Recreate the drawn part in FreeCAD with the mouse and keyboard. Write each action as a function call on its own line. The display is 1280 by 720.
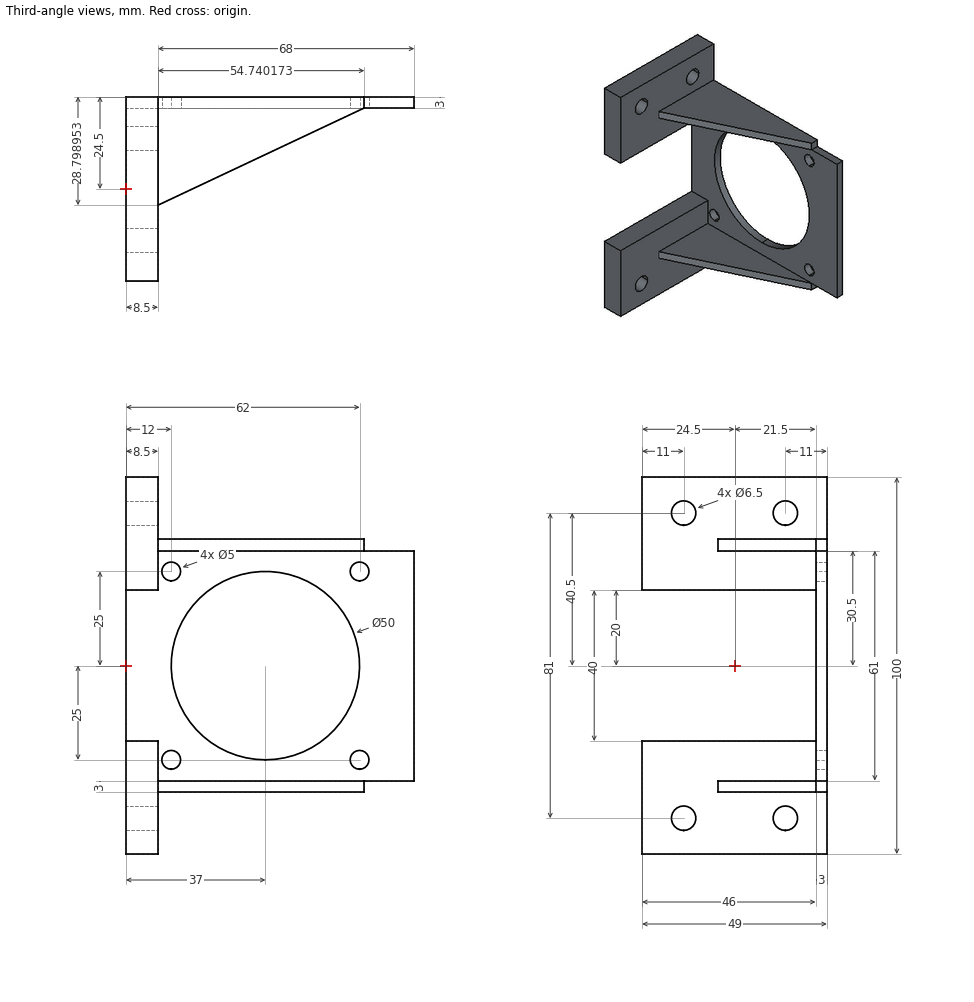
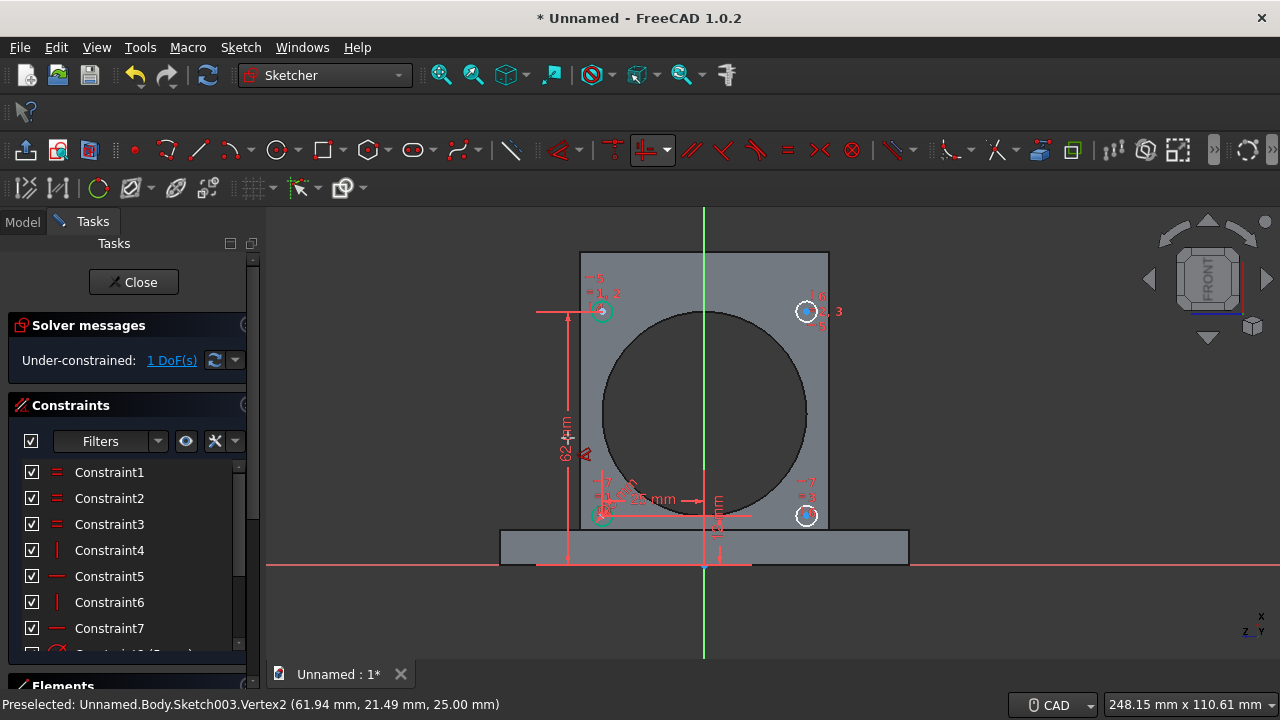
click(807, 312)
click(756, 599)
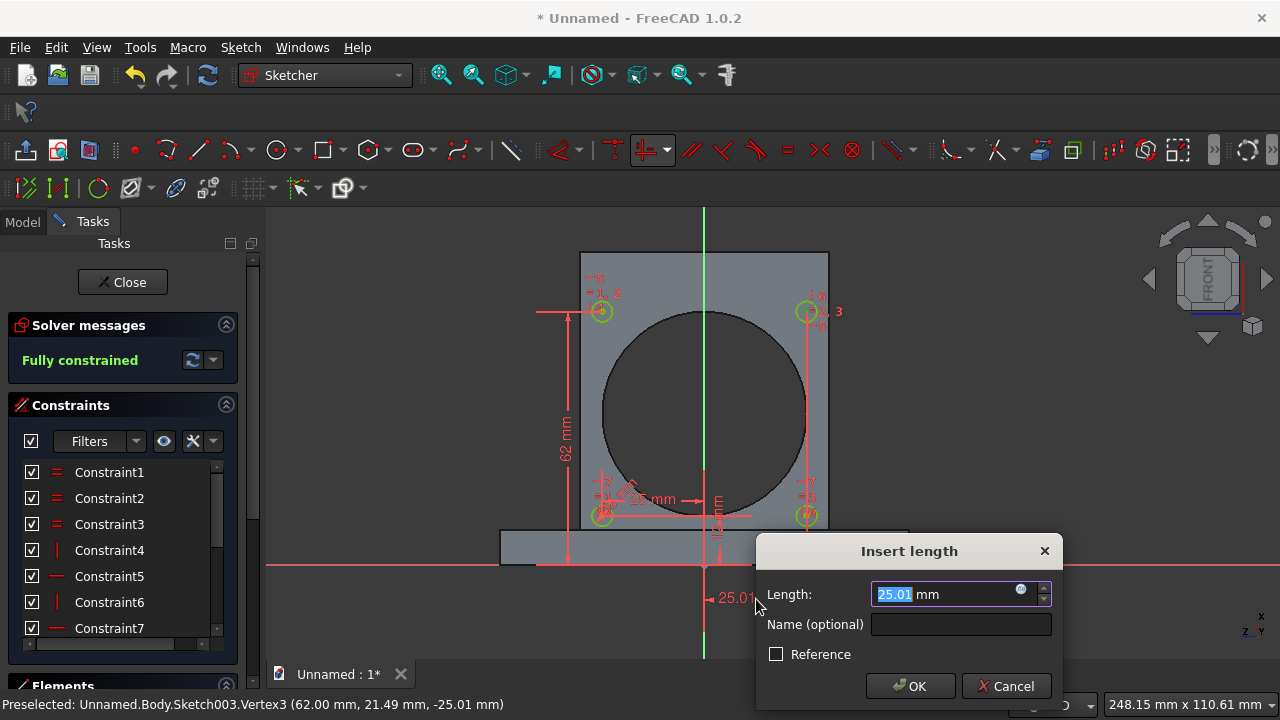
text(25)
key(Return)
key(Escape)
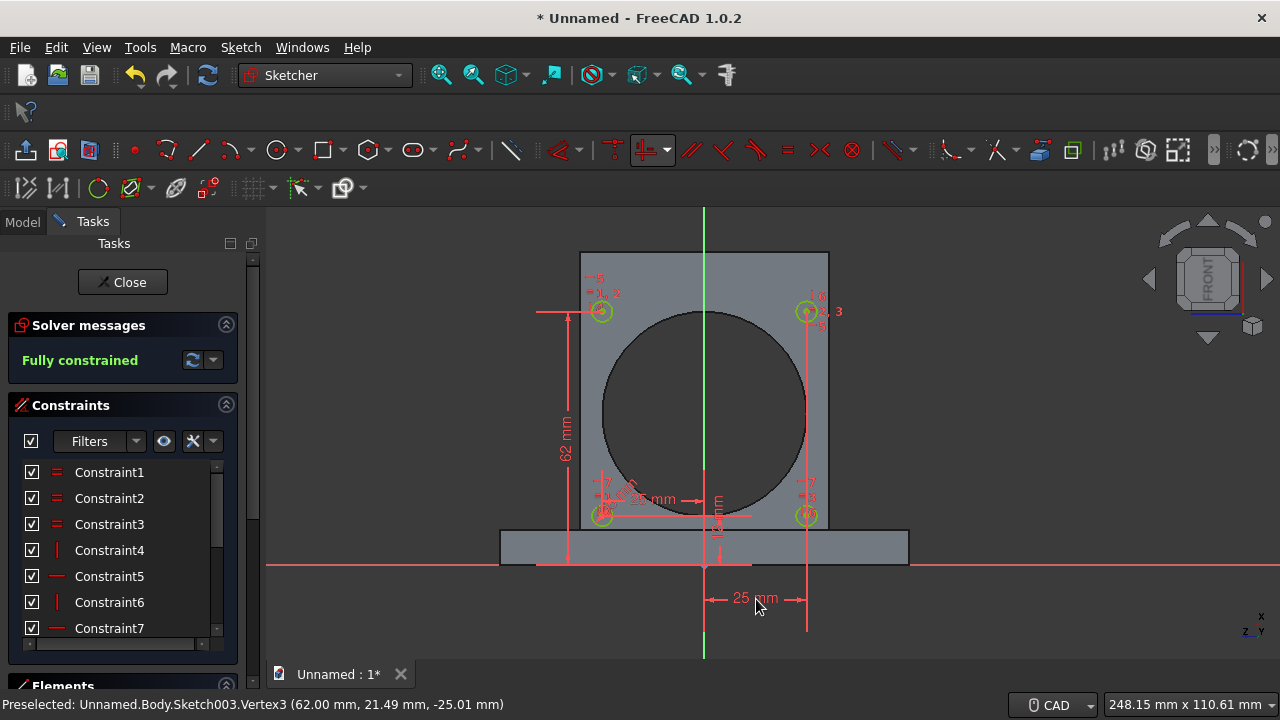
click(123, 282)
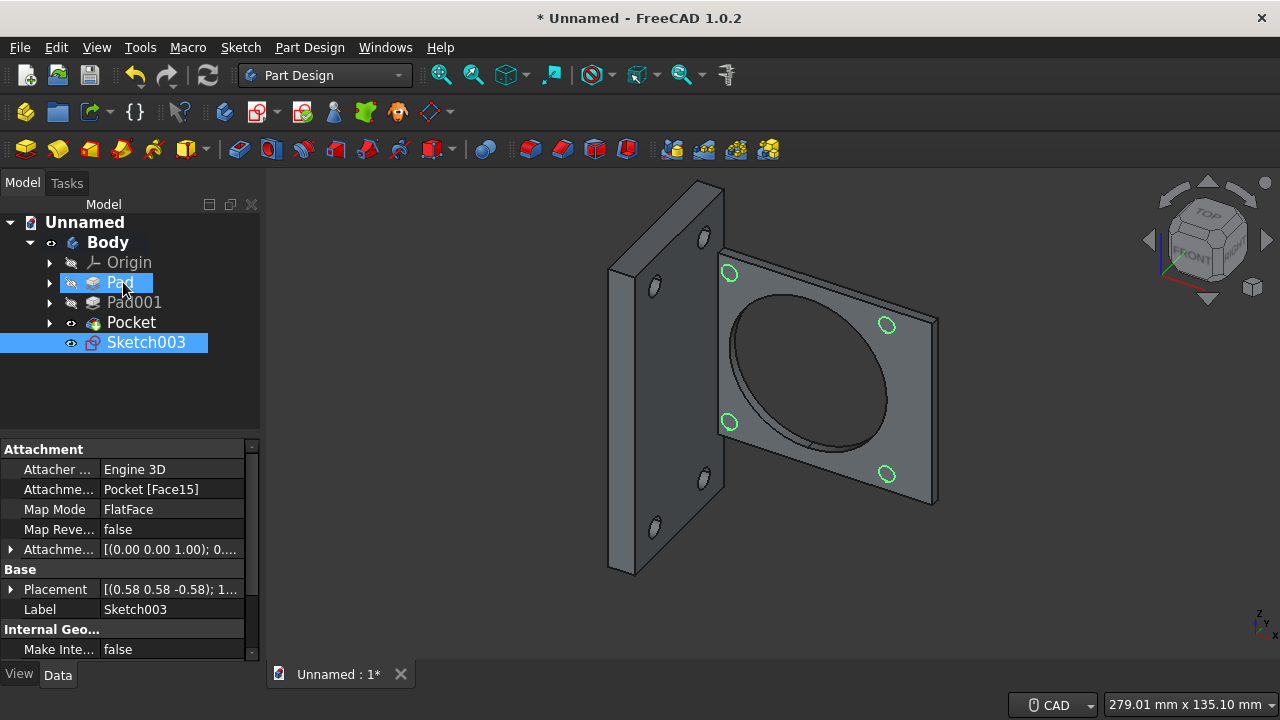
click(240, 150)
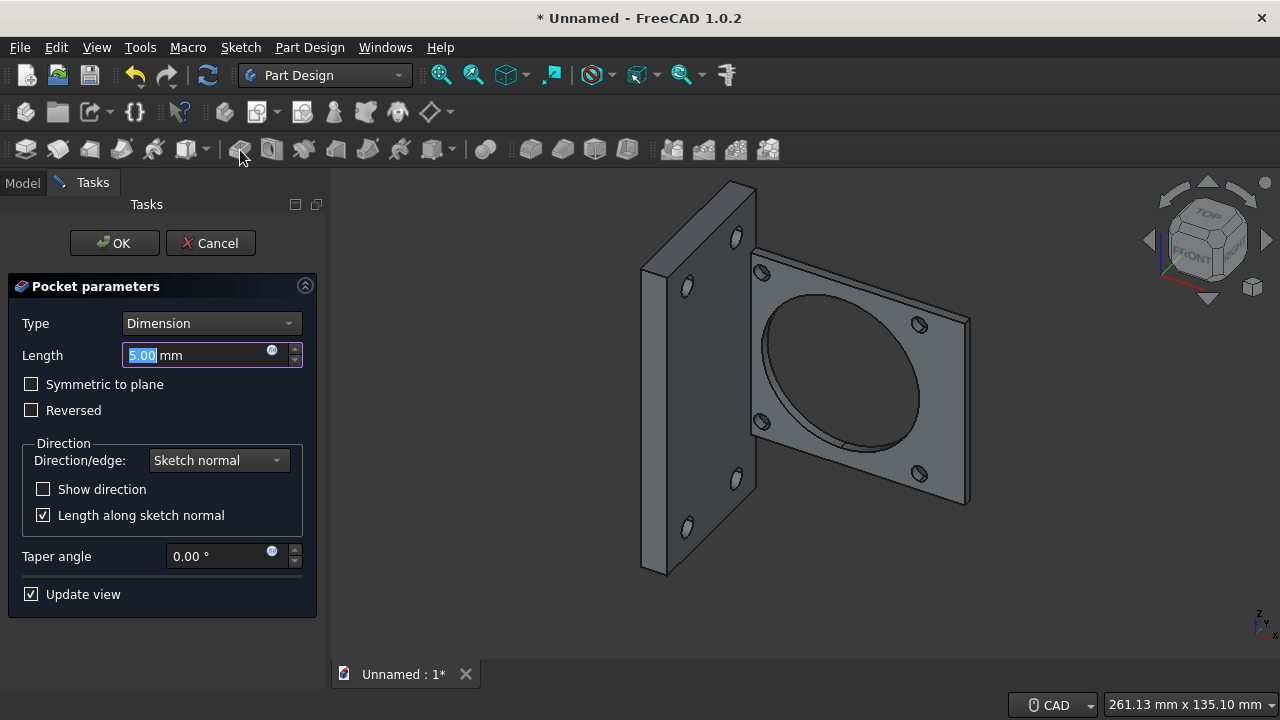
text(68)
key(Tab)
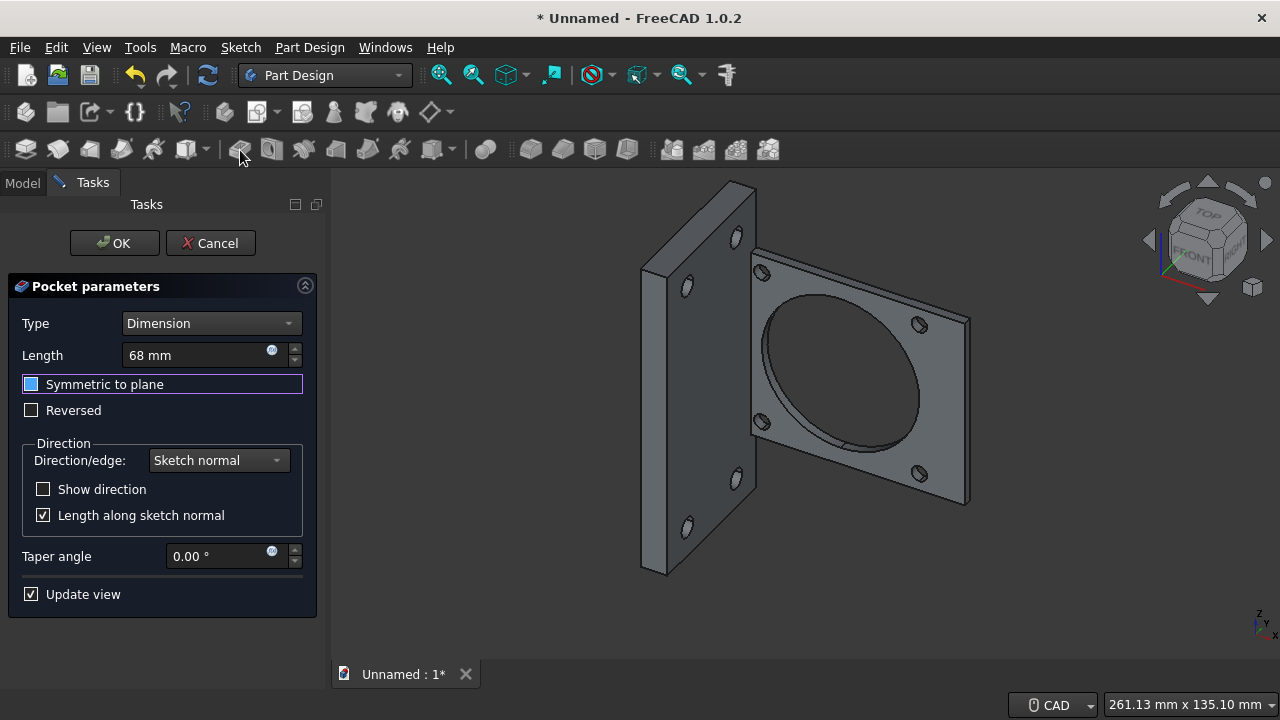
click(115, 243)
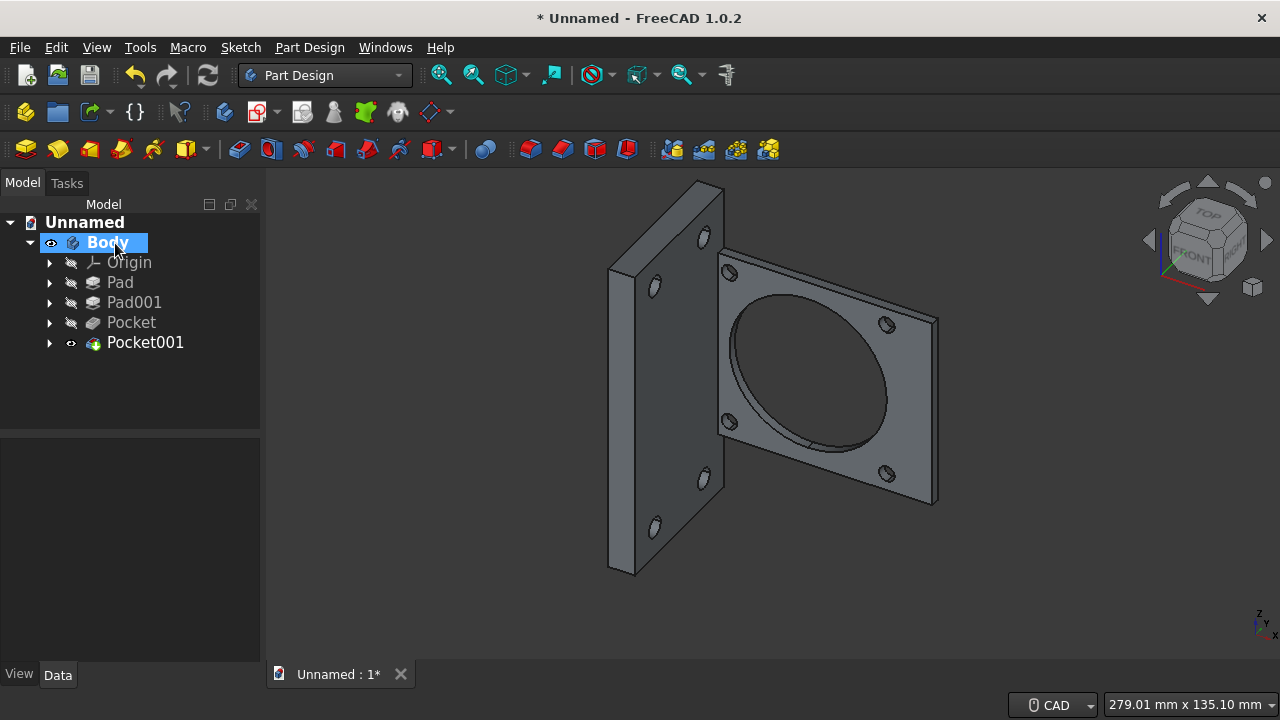
click(679, 424)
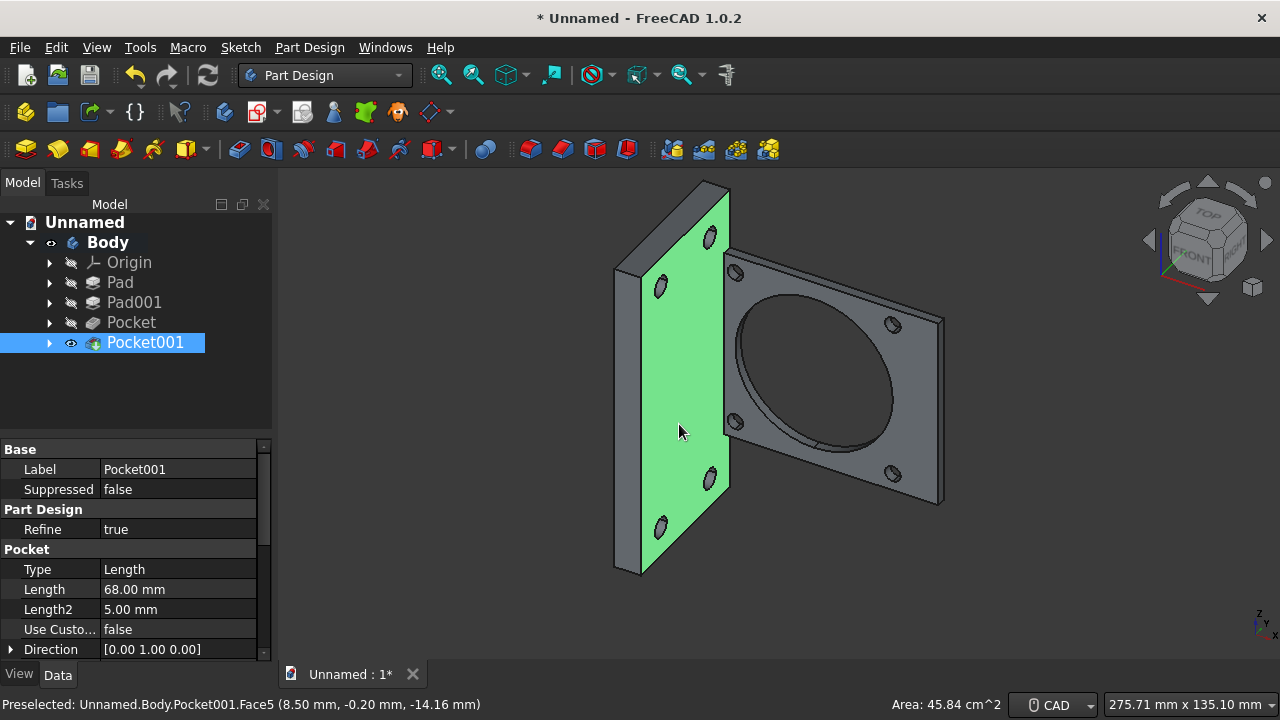
click(258, 112)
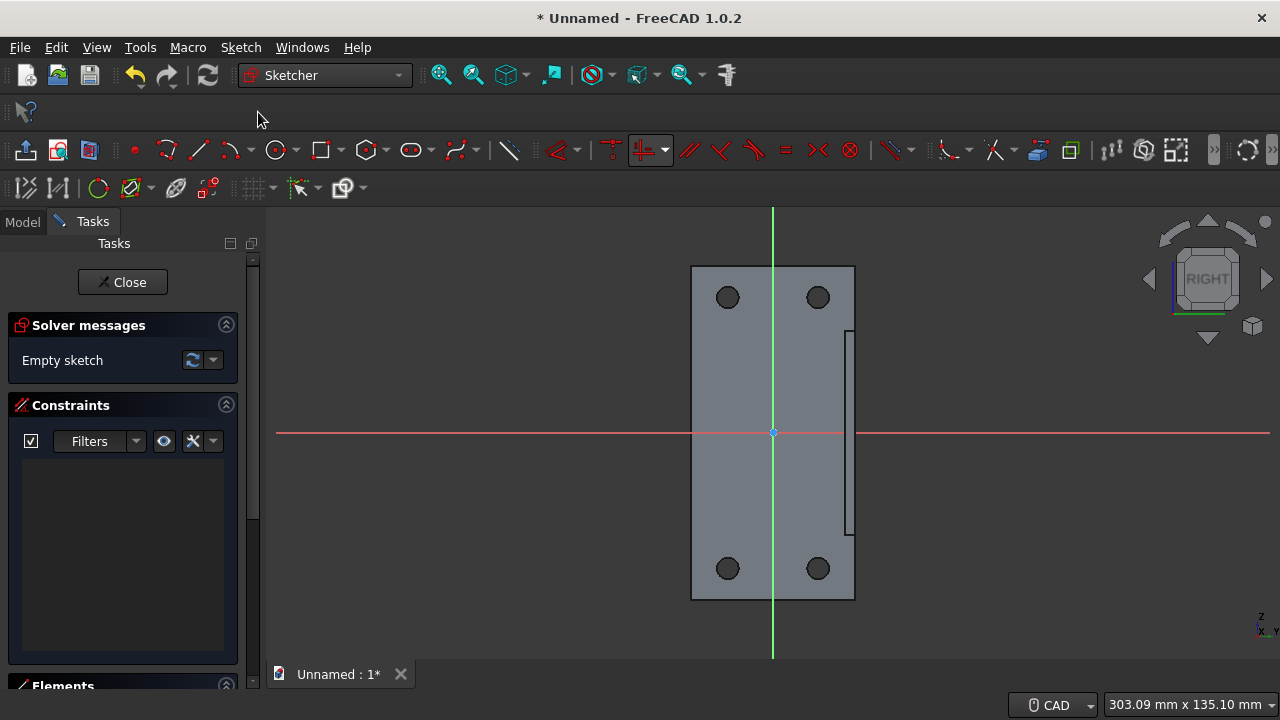
click(90, 150)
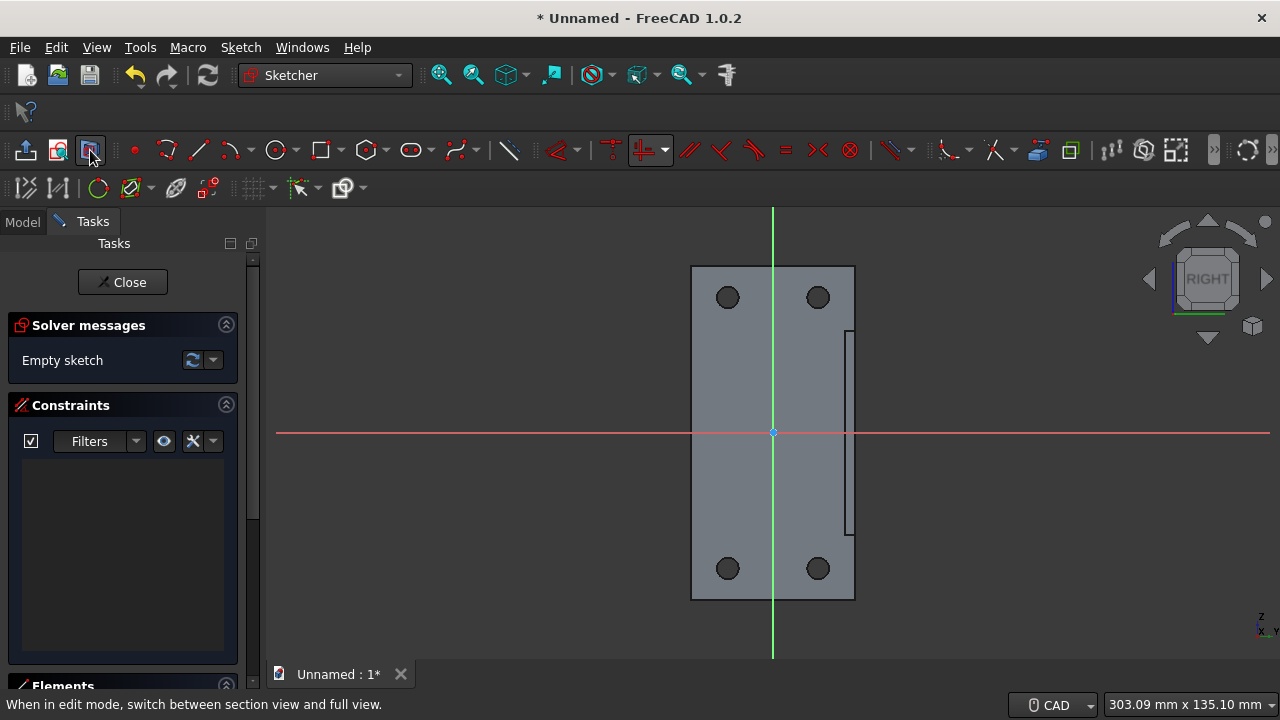
scroll(820, 433, up, 4)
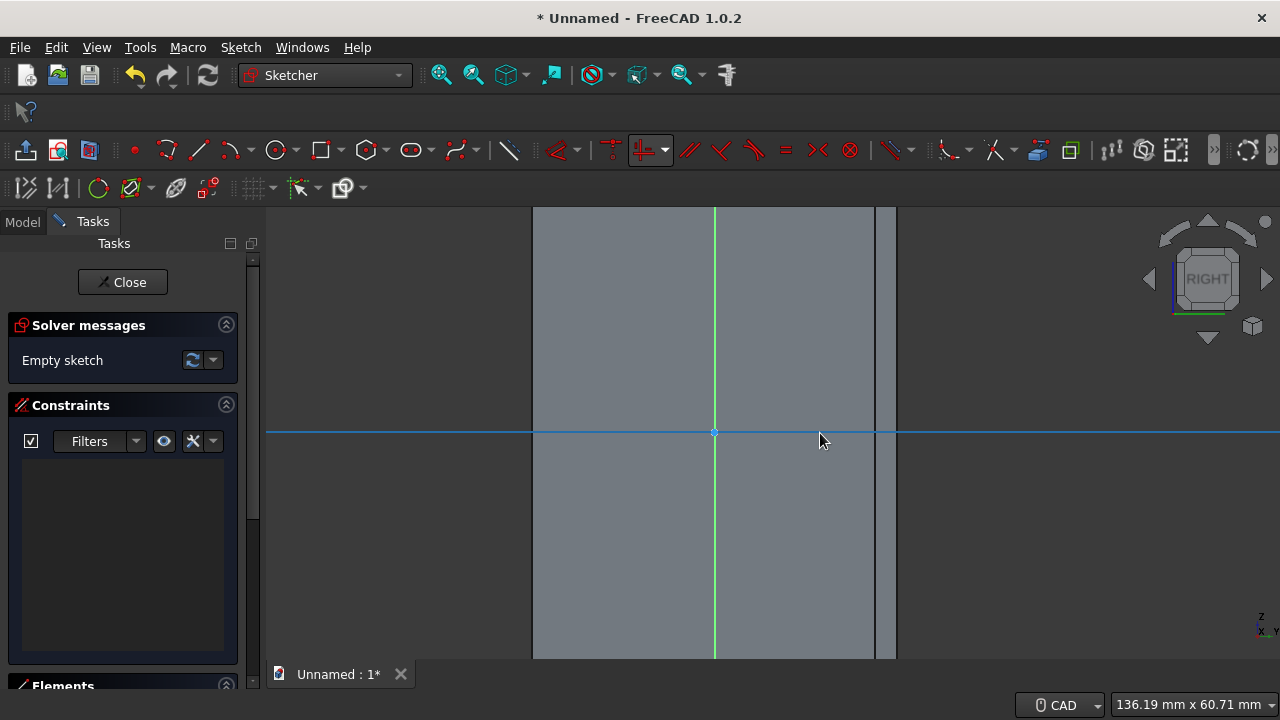
key(g)
key(r)